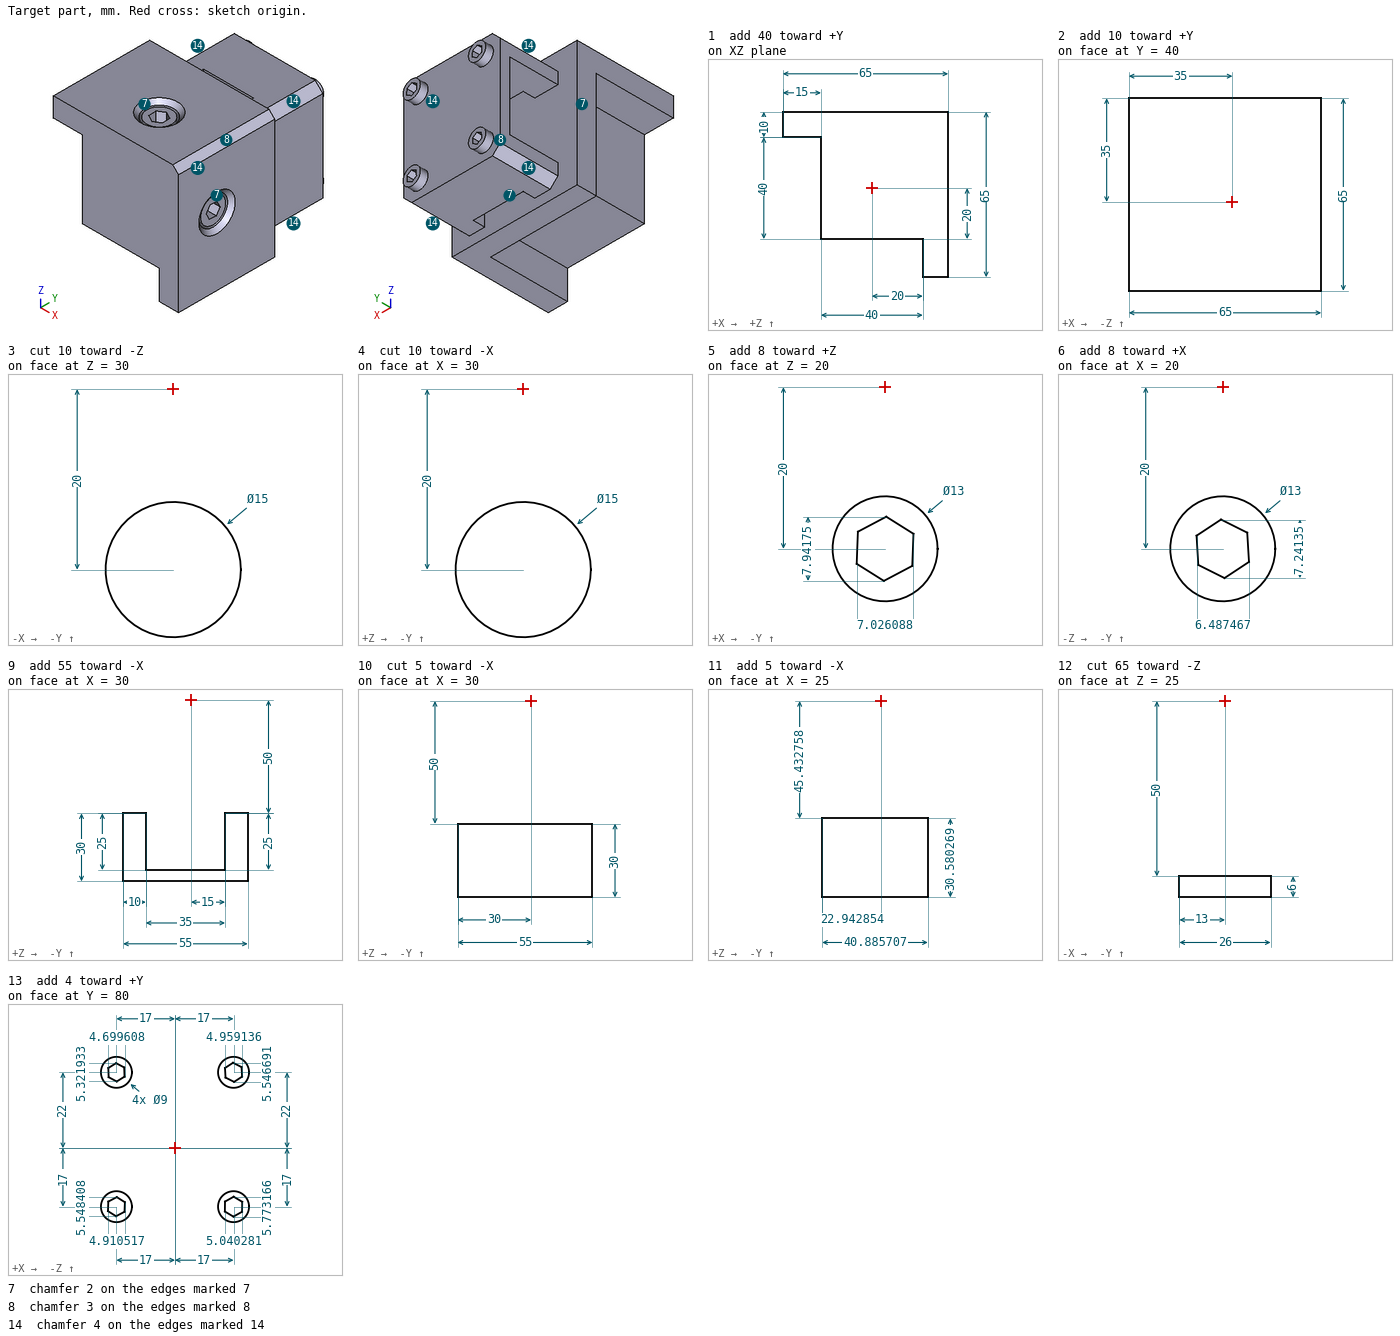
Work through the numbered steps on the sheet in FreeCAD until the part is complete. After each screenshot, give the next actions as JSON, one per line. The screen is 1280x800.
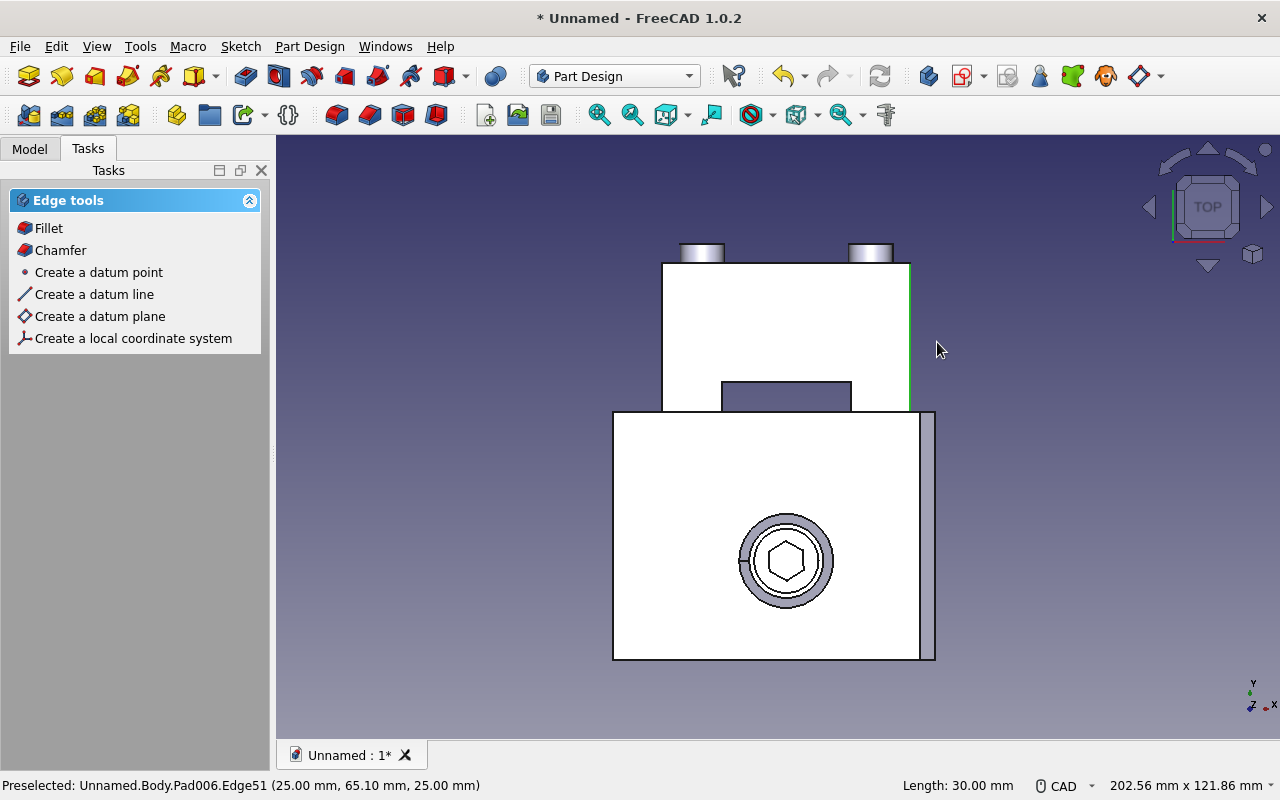
{"action": "left_click", "coordinate": [662, 337], "text": "ctrl"}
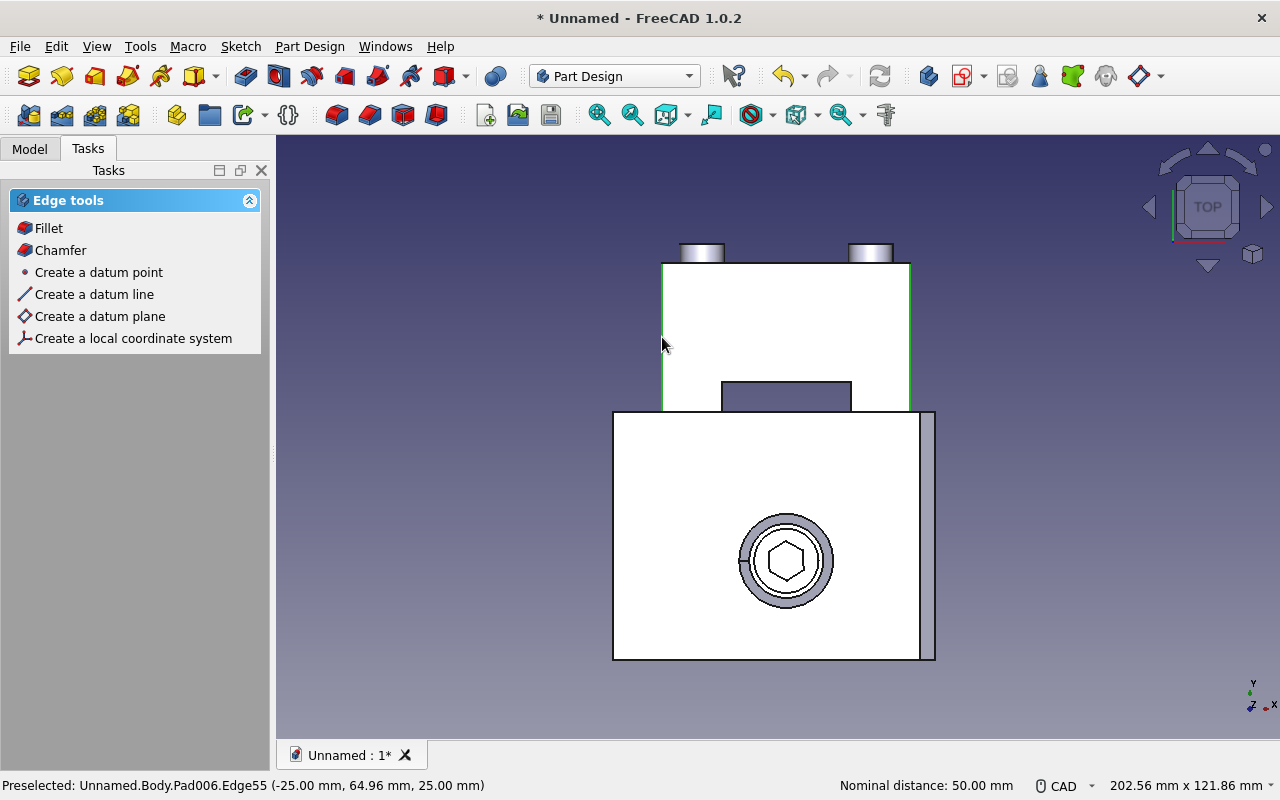
{"action": "key", "text": "1"}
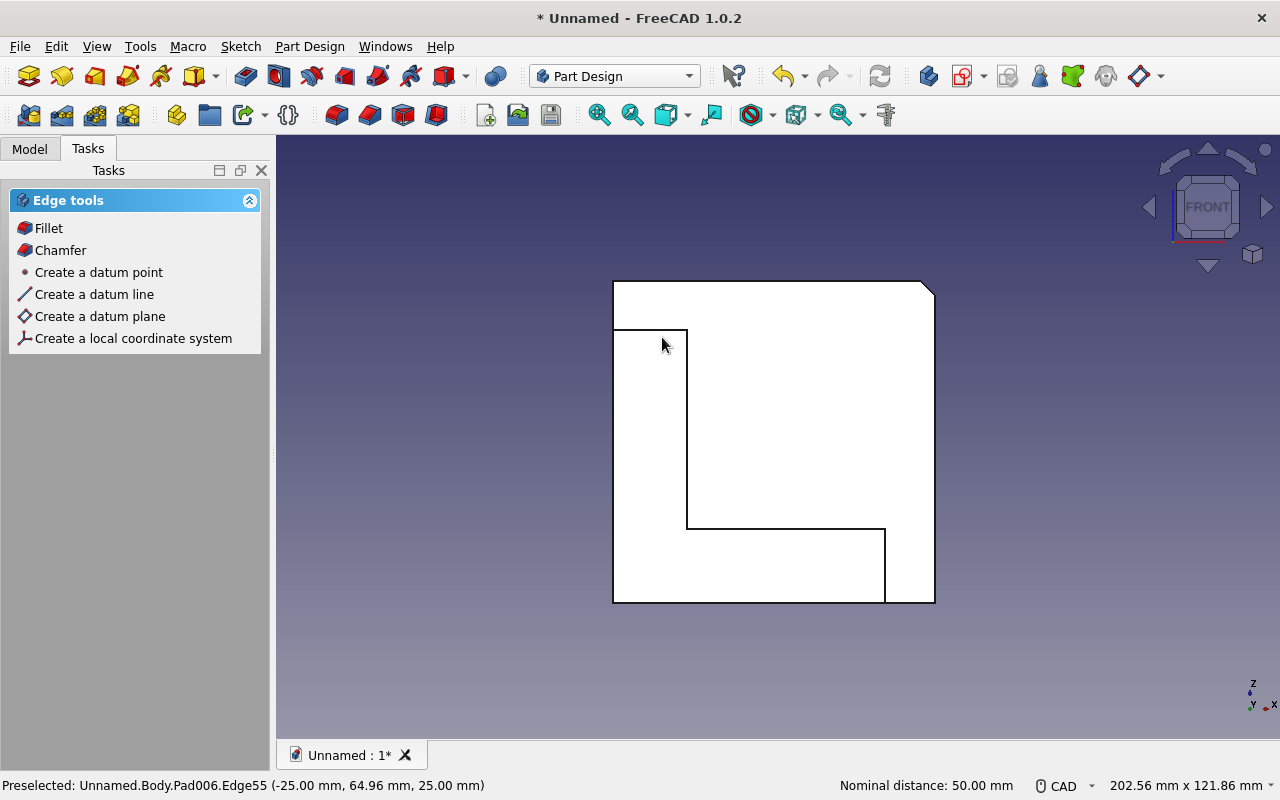
{"action": "key", "text": "3"}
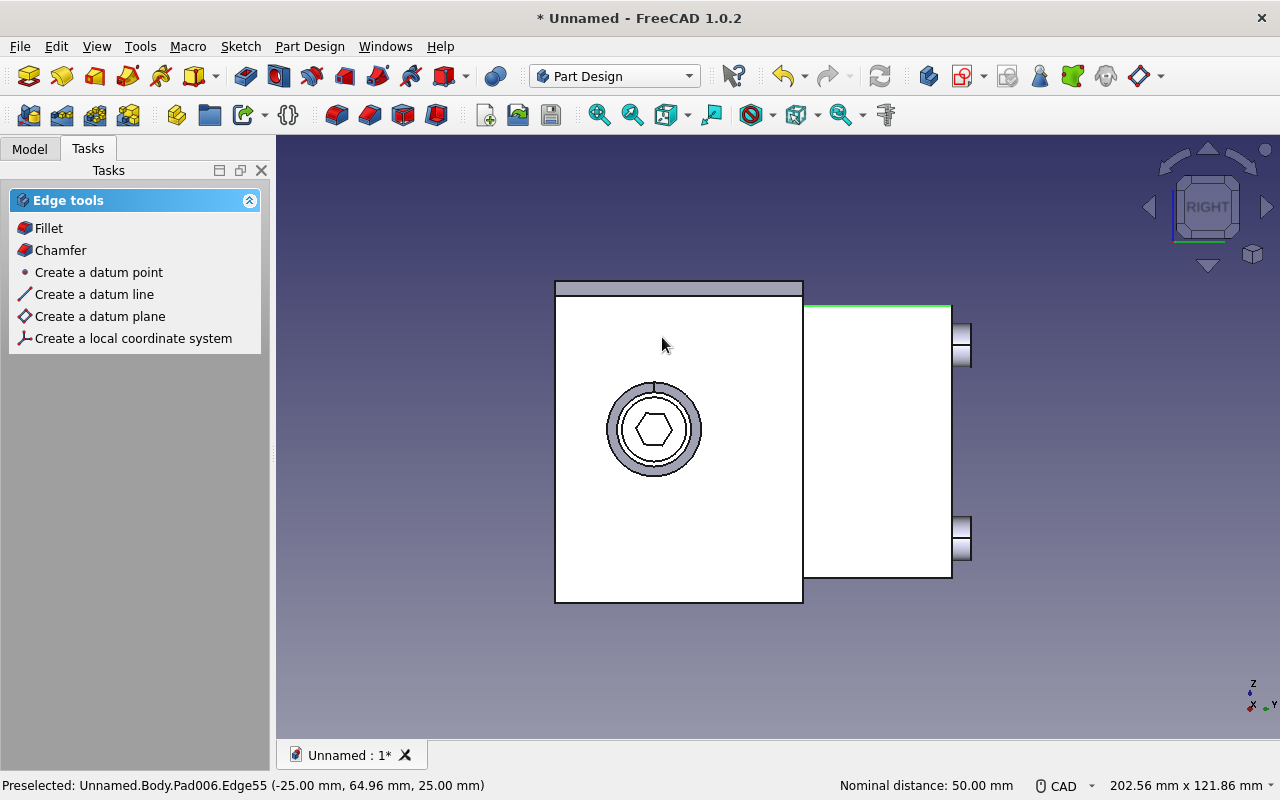
{"action": "left_click", "coordinate": [877, 577], "text": "ctrl"}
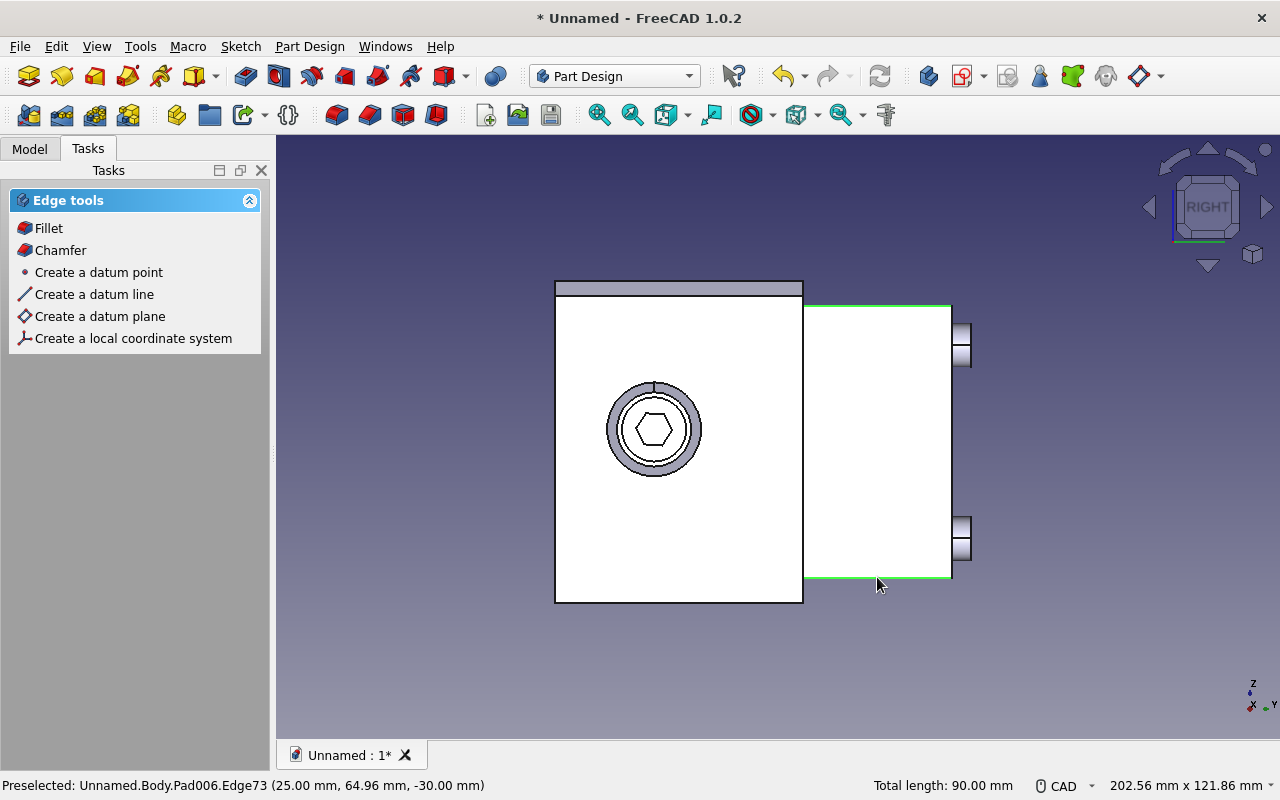
{"action": "key", "text": "5"}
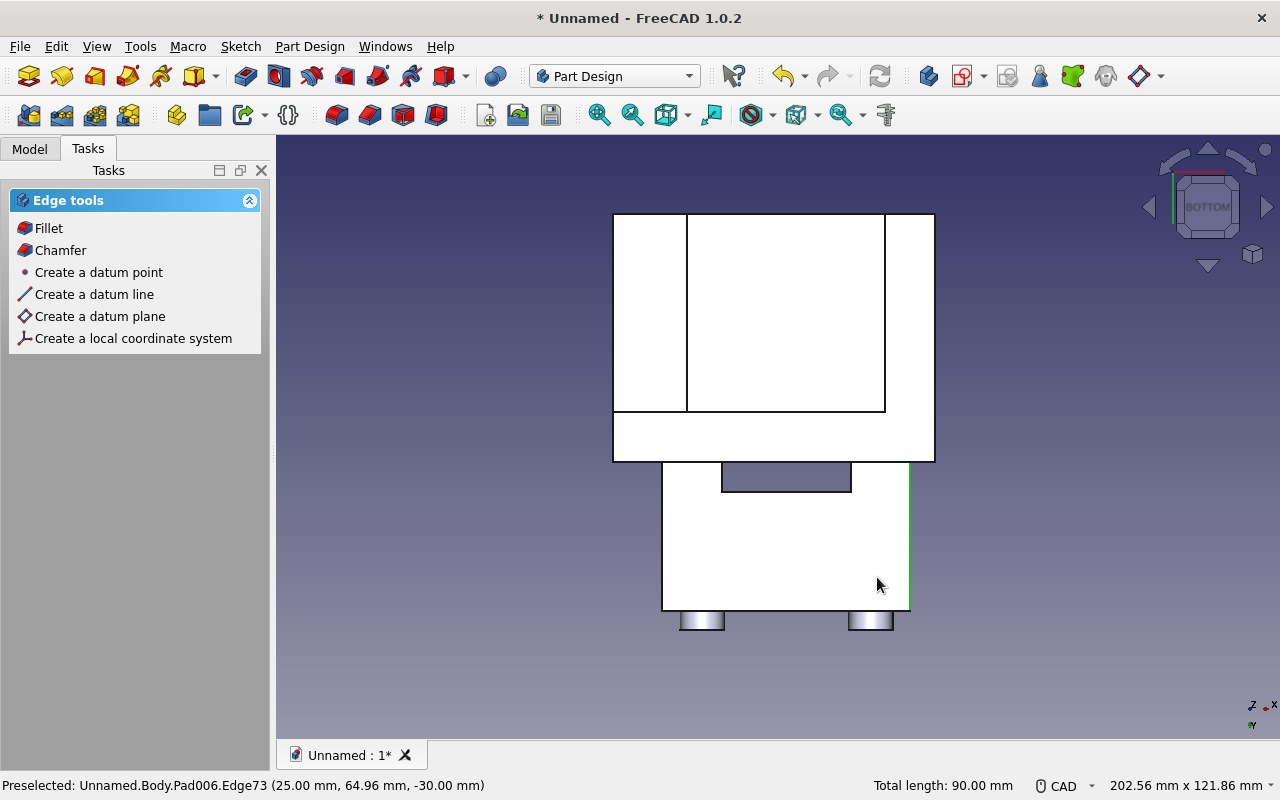
{"action": "left_click", "coordinate": [662, 535], "text": "ctrl"}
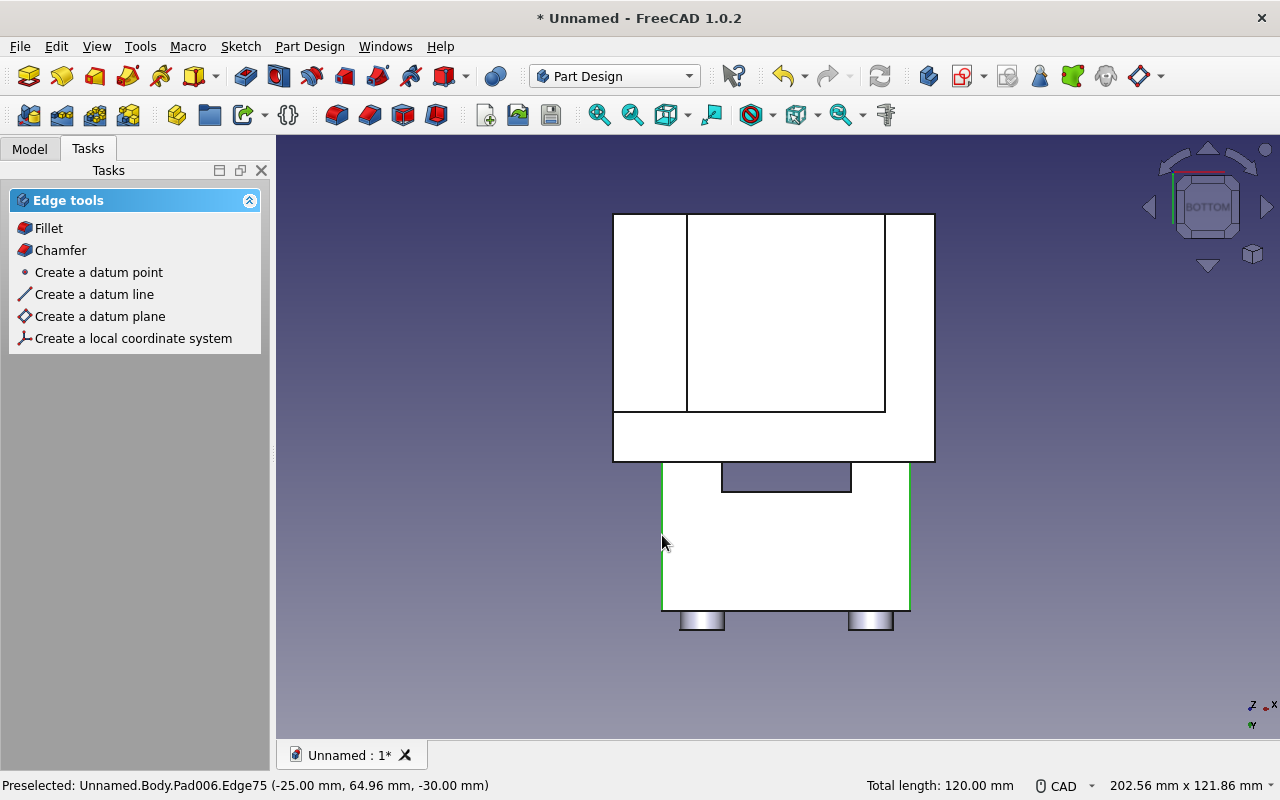
{"action": "left_click", "coordinate": [370, 116]}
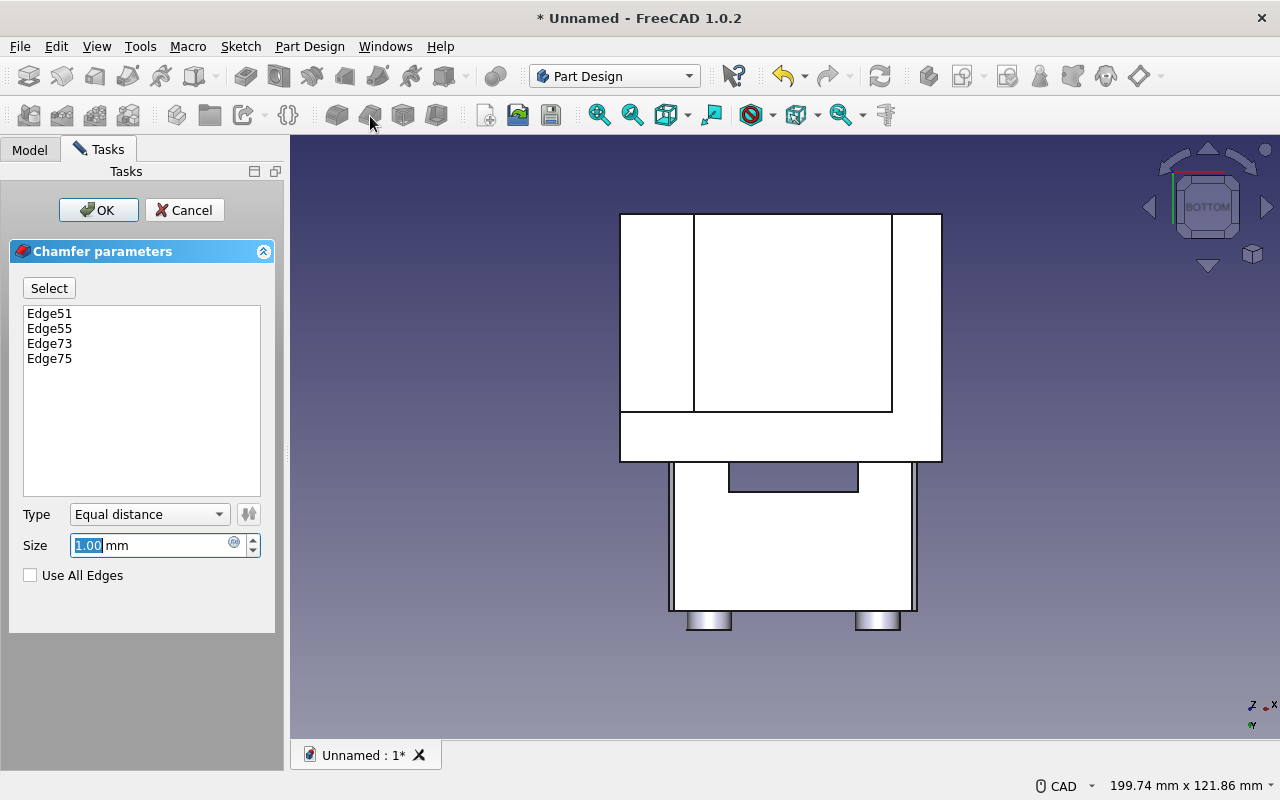
{"action": "type", "text": "4"}
{"action": "key", "text": "Tab"}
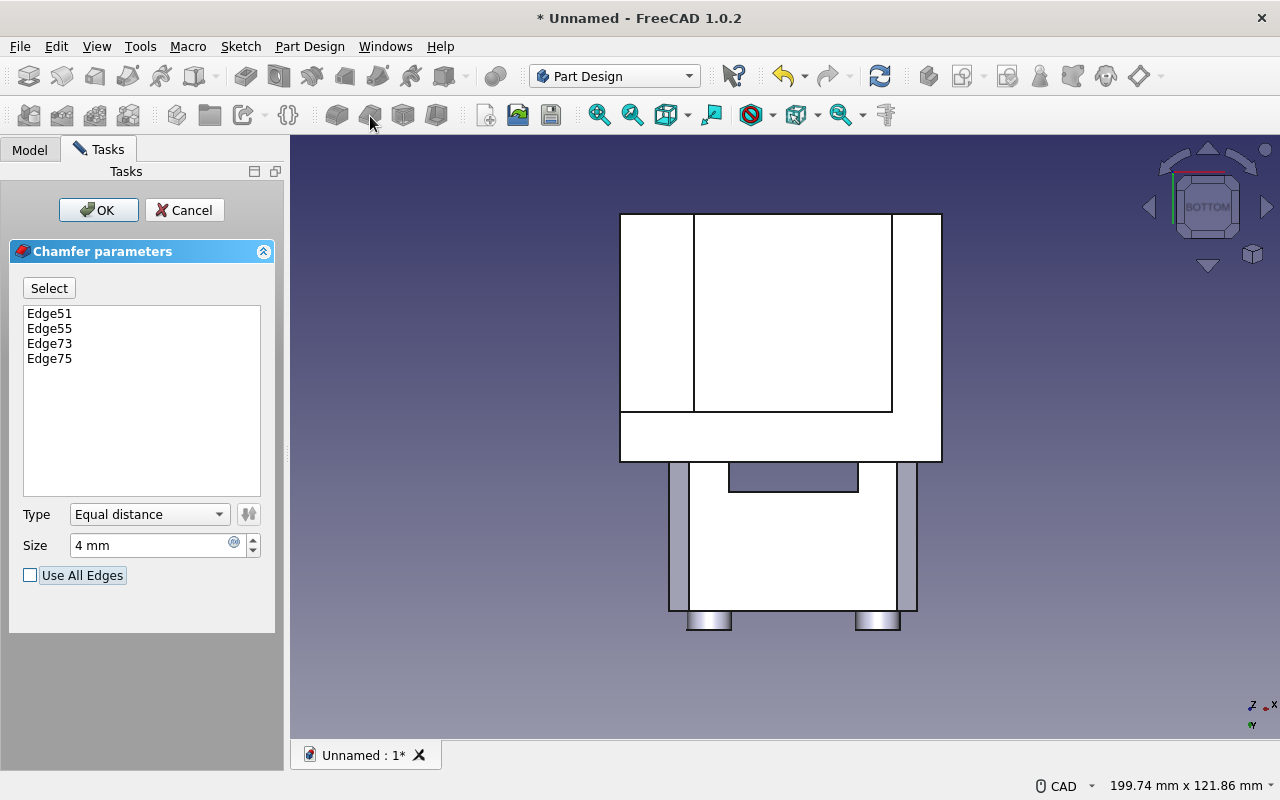
{"action": "left_click", "coordinate": [99, 210]}